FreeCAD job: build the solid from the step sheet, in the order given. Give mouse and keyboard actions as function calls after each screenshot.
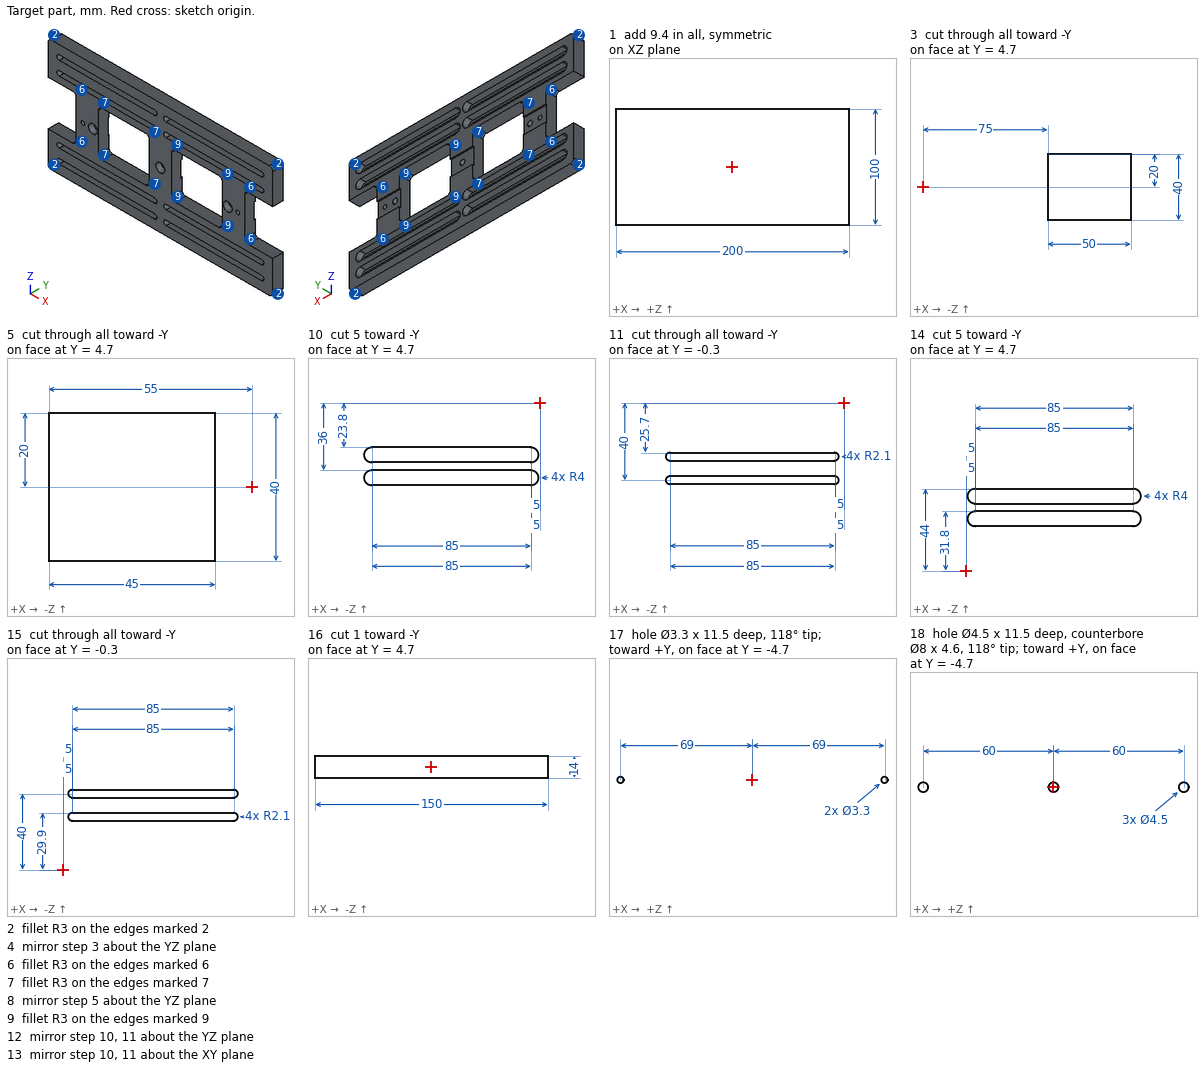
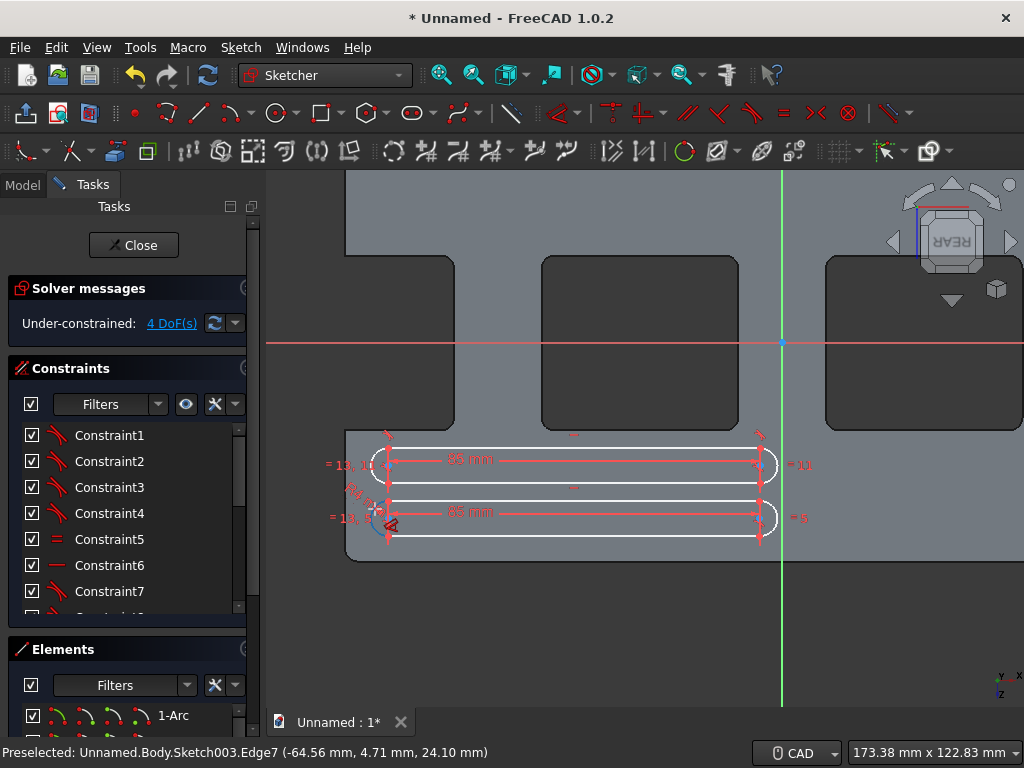
scroll(760, 536, up, 3)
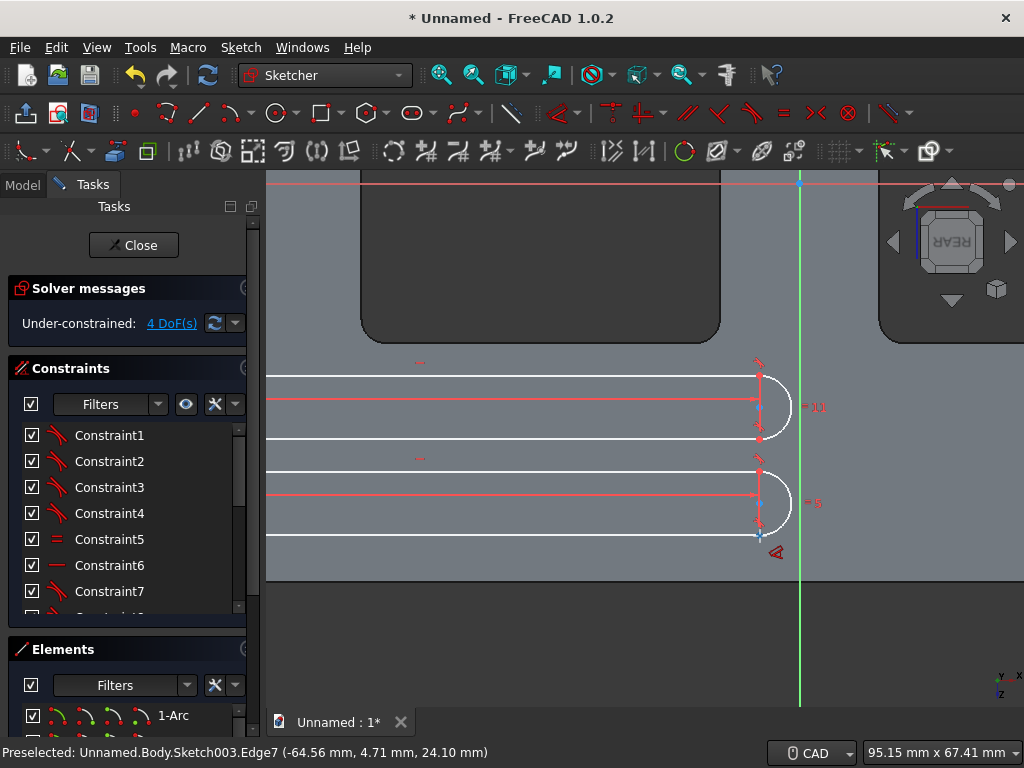
click(759, 535)
click(780, 569)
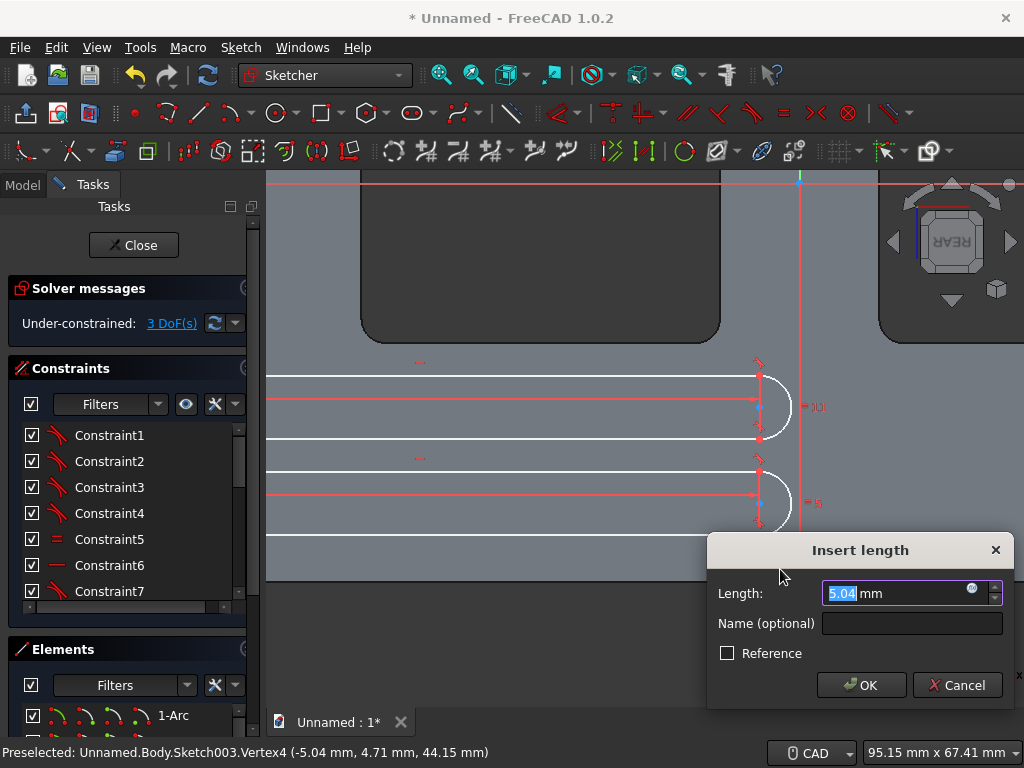
text(5)
key(Return)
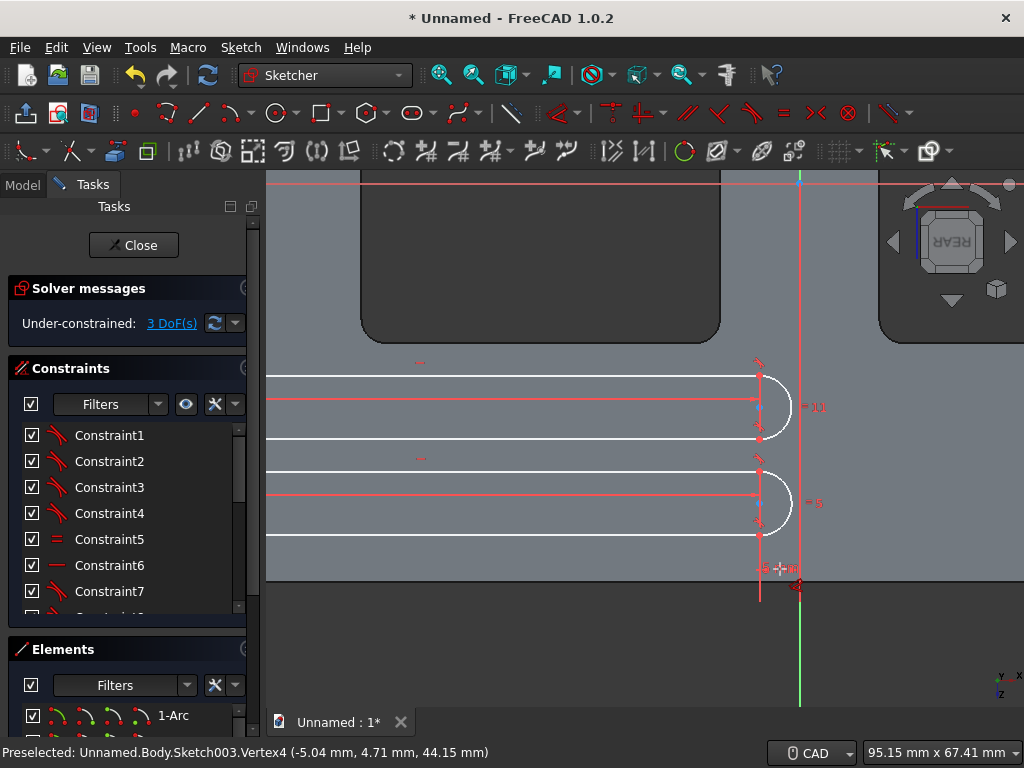
click(760, 439)
click(770, 497)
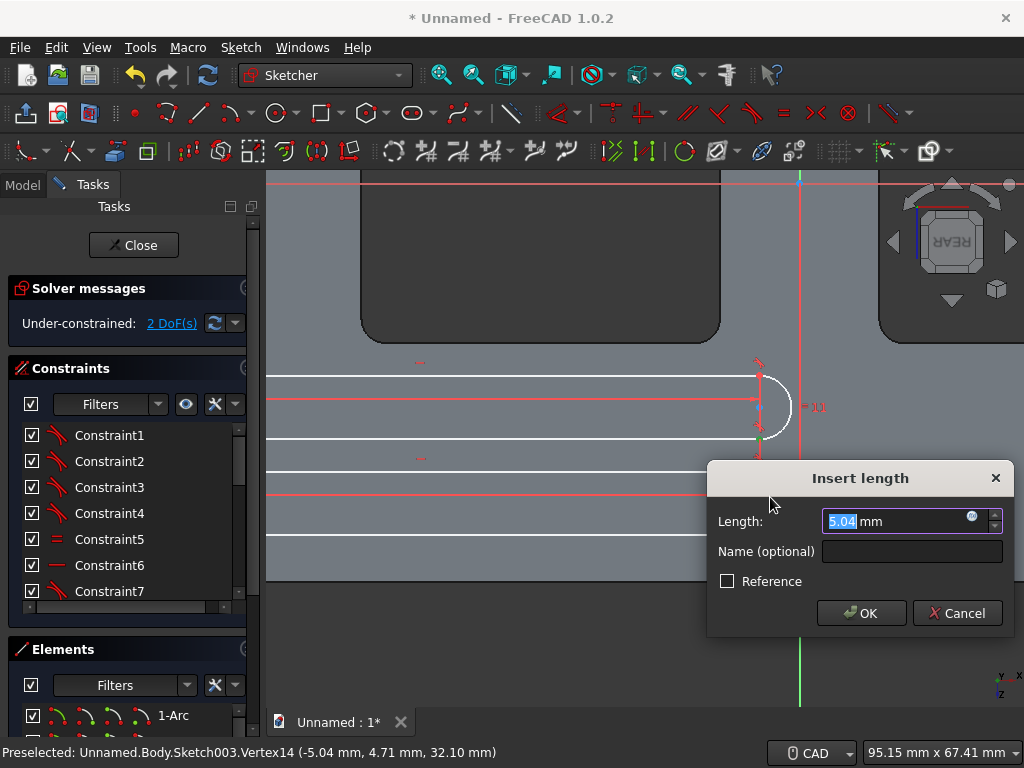
text(5)
key(Return)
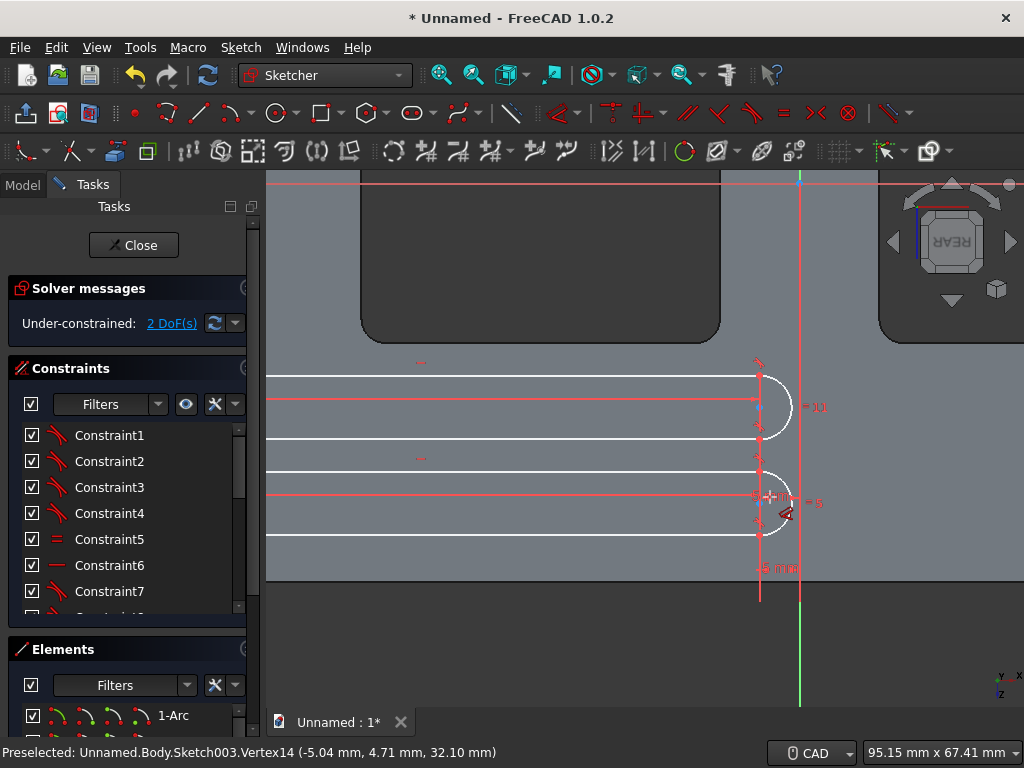
scroll(761, 535, down, 3)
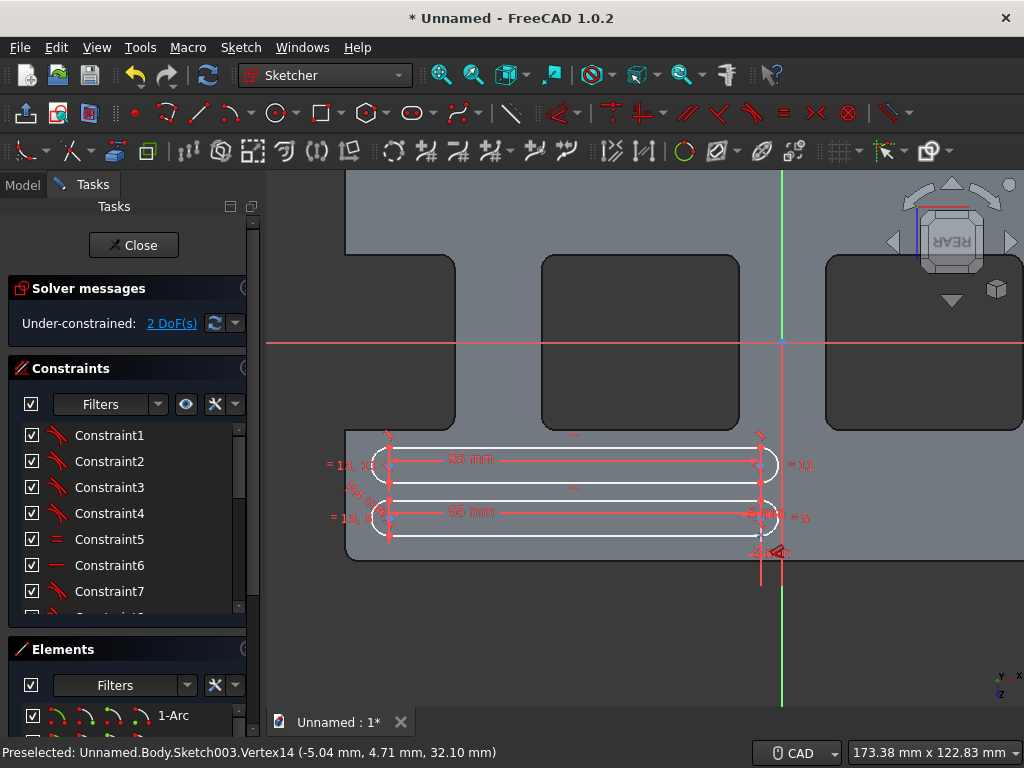
click(389, 501)
click(816, 422)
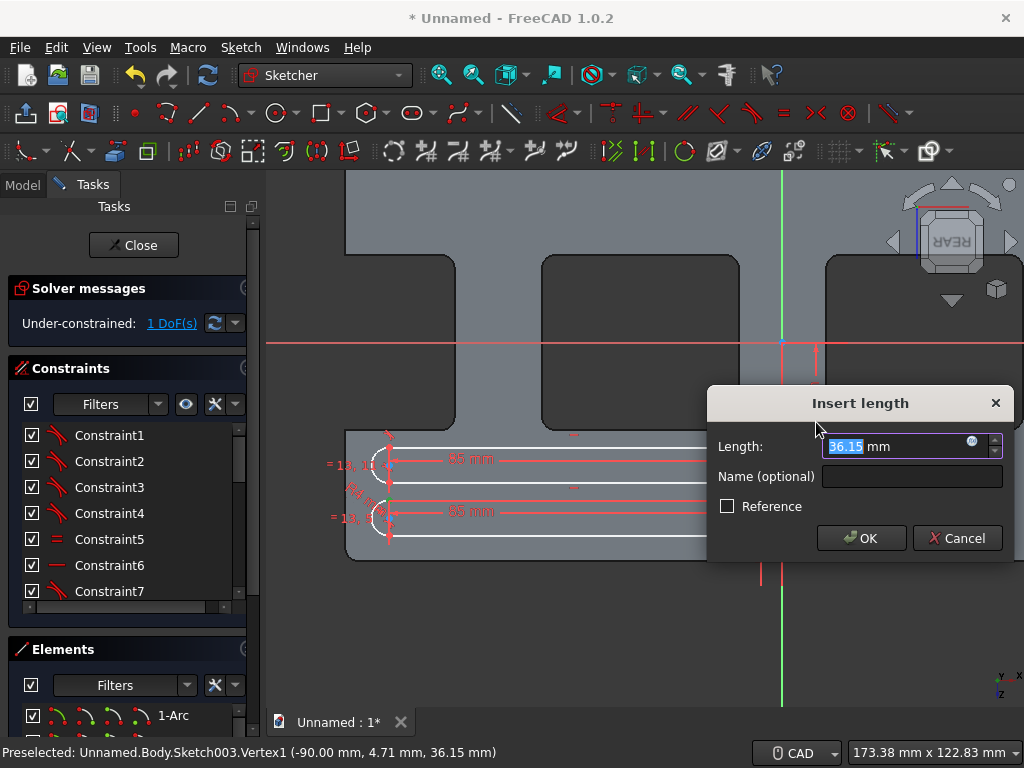
text(36)
key(Return)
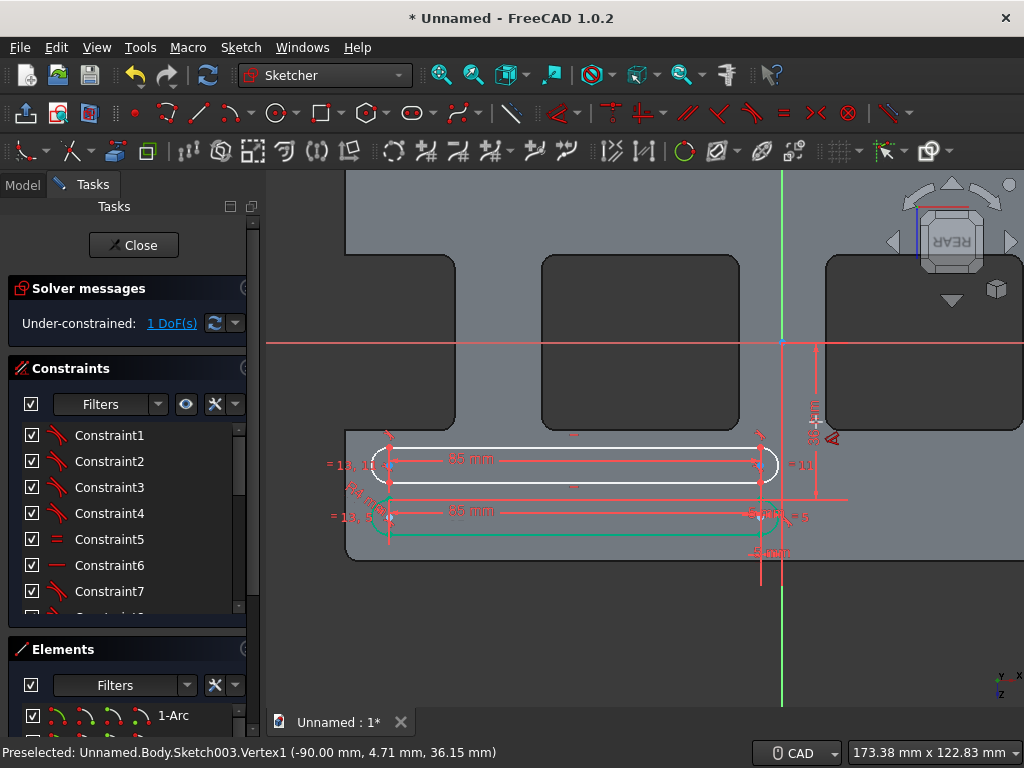
click(389, 448)
click(816, 395)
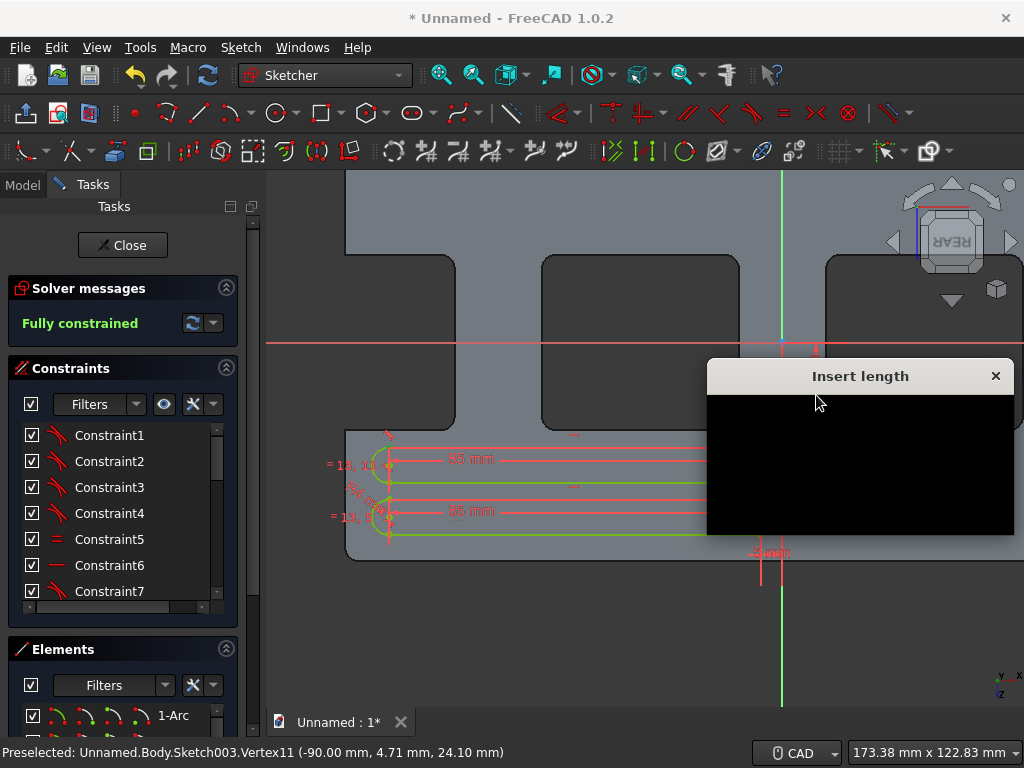
text(23.8)
key(Return)
key(Escape)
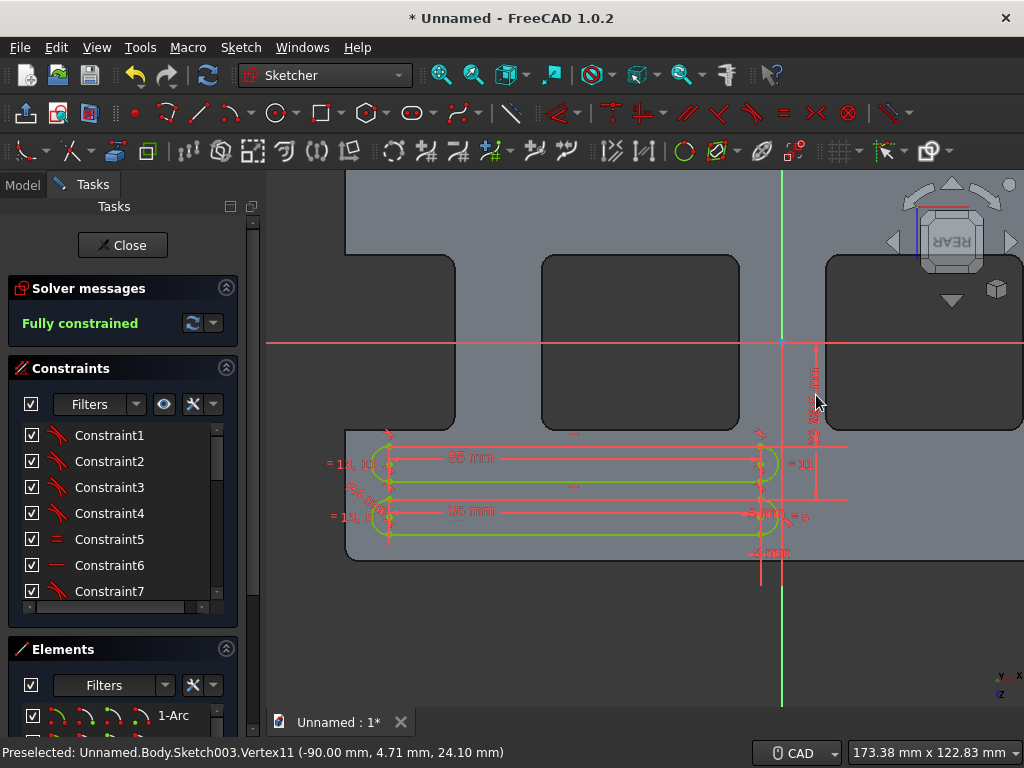
click(123, 245)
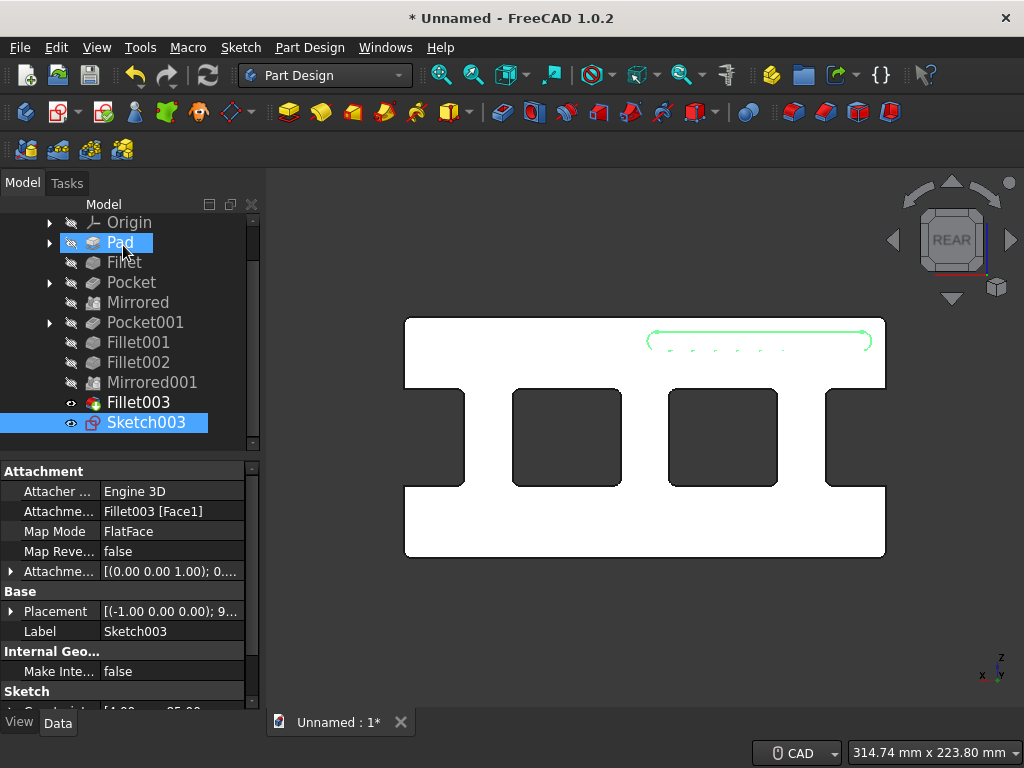
click(504, 112)